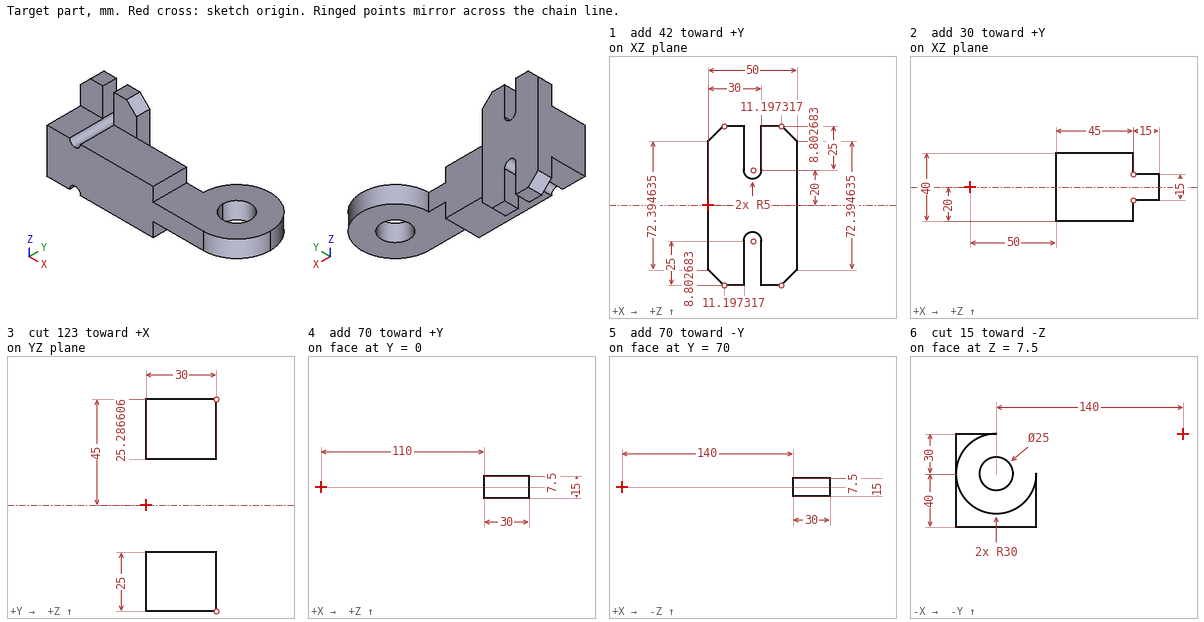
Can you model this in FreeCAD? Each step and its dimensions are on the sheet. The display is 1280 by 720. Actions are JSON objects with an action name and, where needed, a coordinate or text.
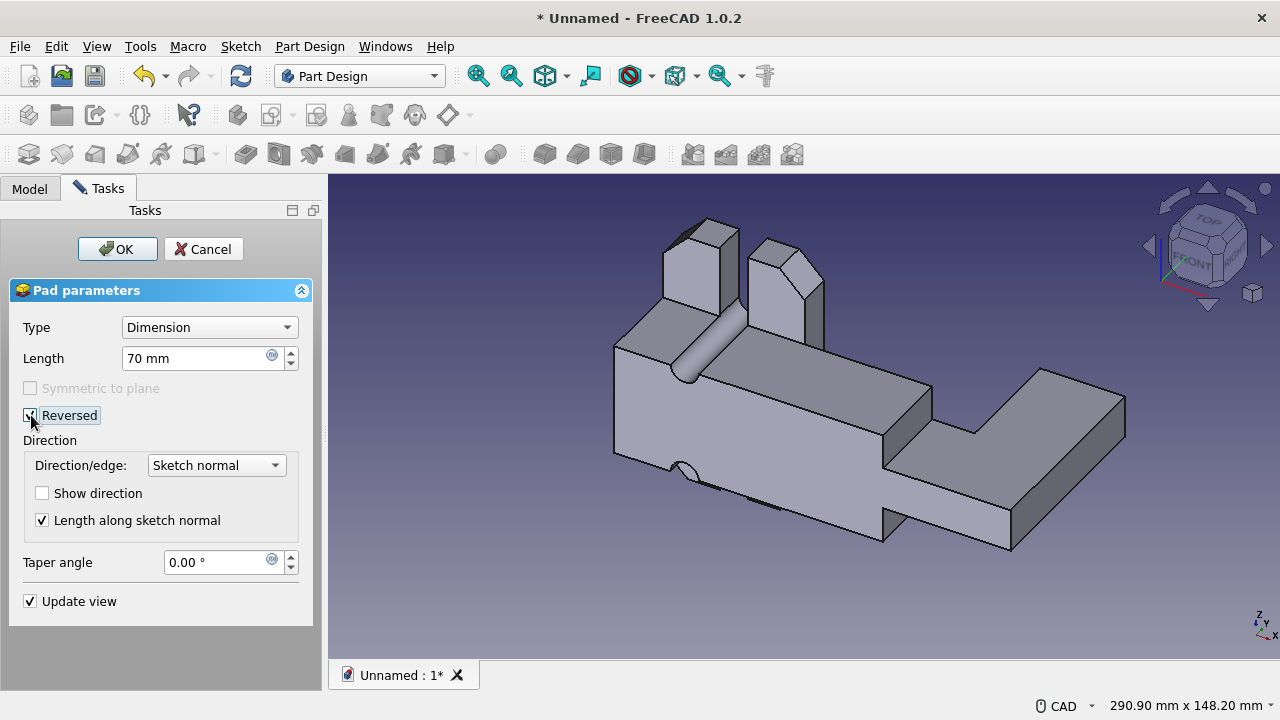
{"action": "left_click", "coordinate": [118, 249]}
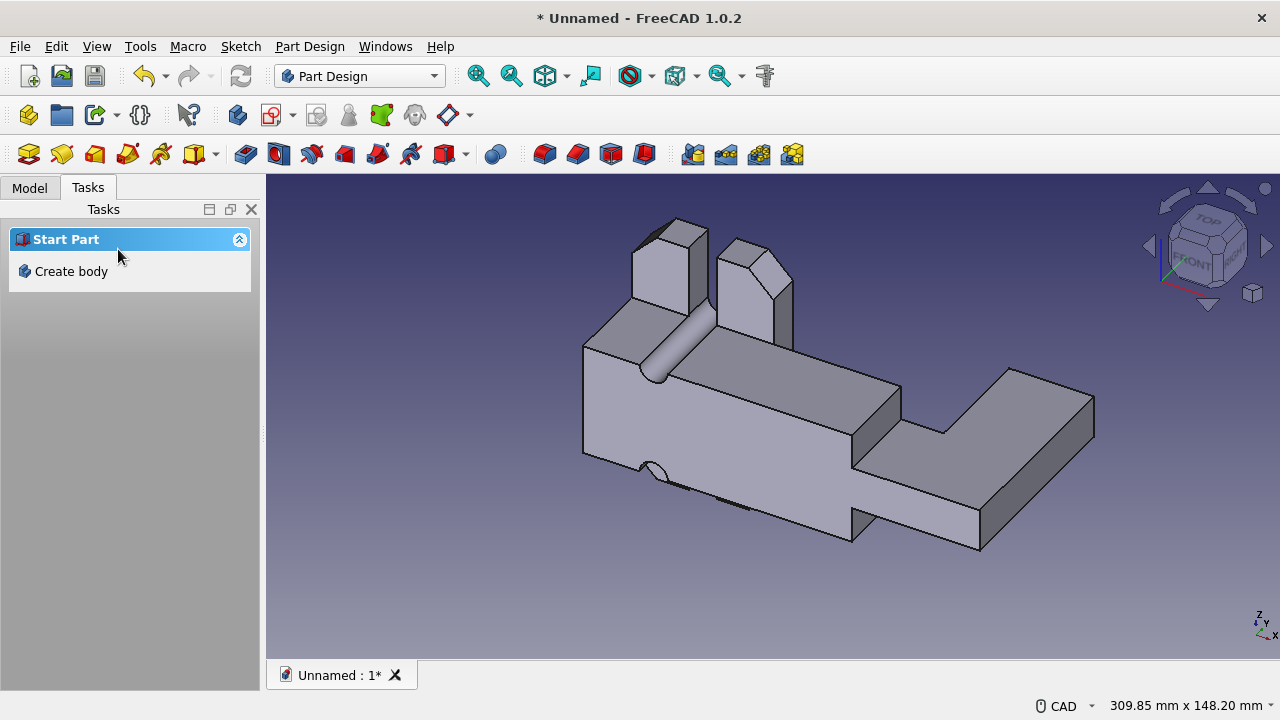
{"action": "left_click", "coordinate": [479, 76]}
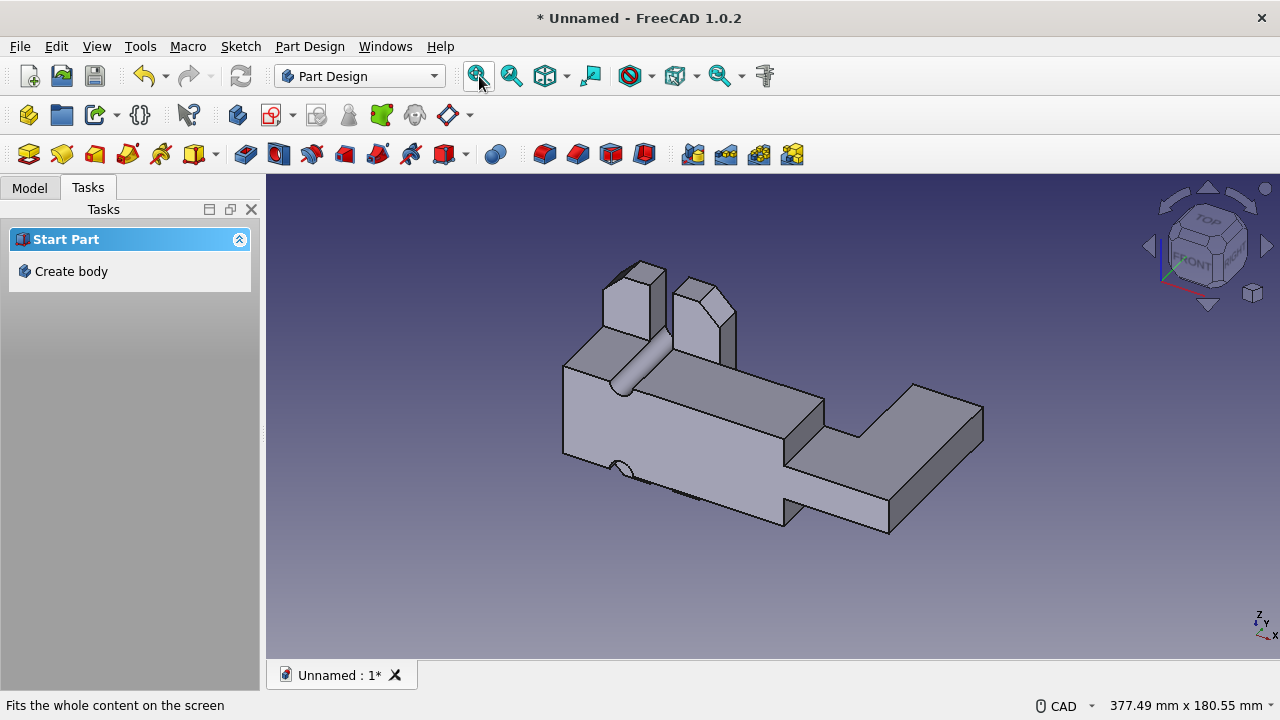
{"action": "key", "text": "4"}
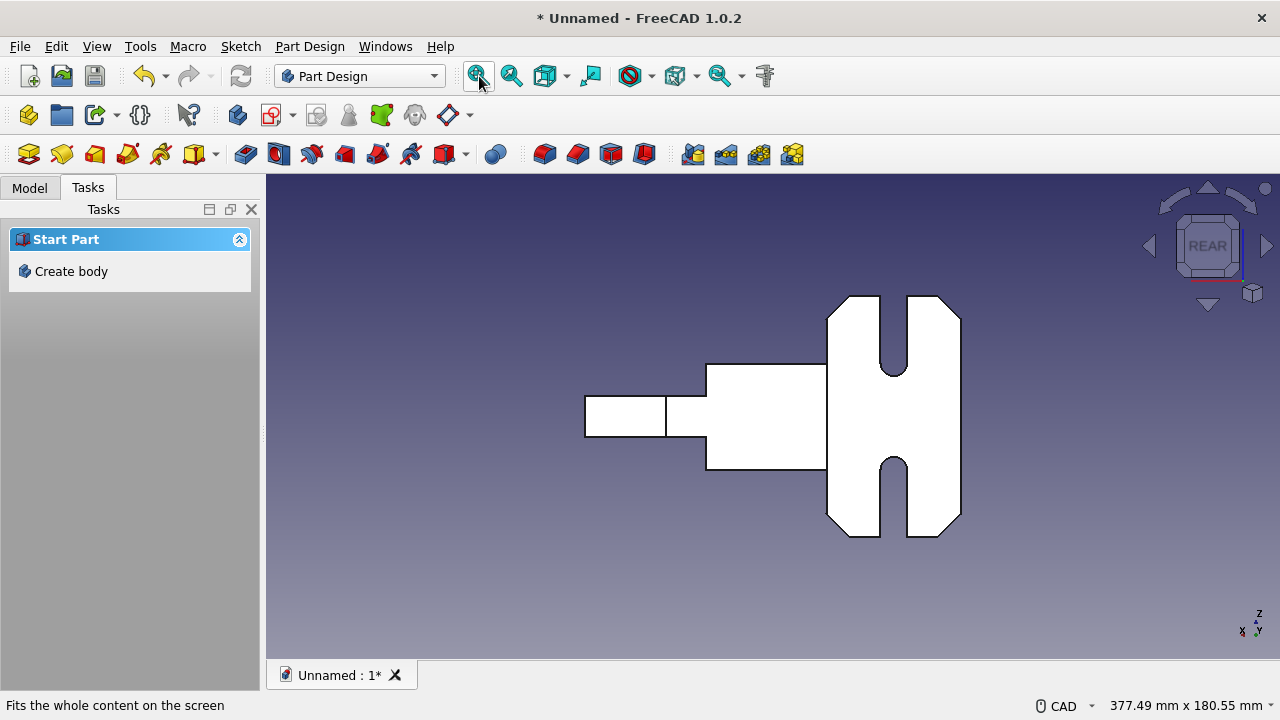
{"action": "left_click", "coordinate": [614, 416]}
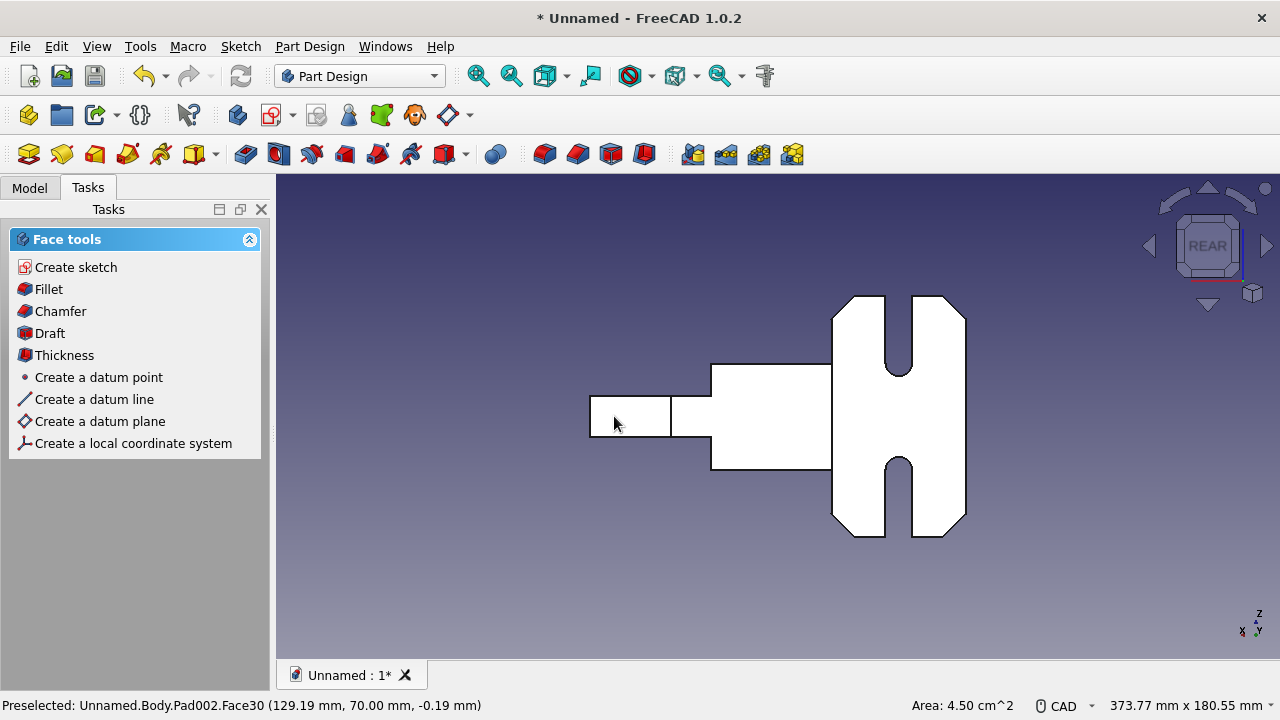
{"action": "left_click", "coordinate": [270, 116]}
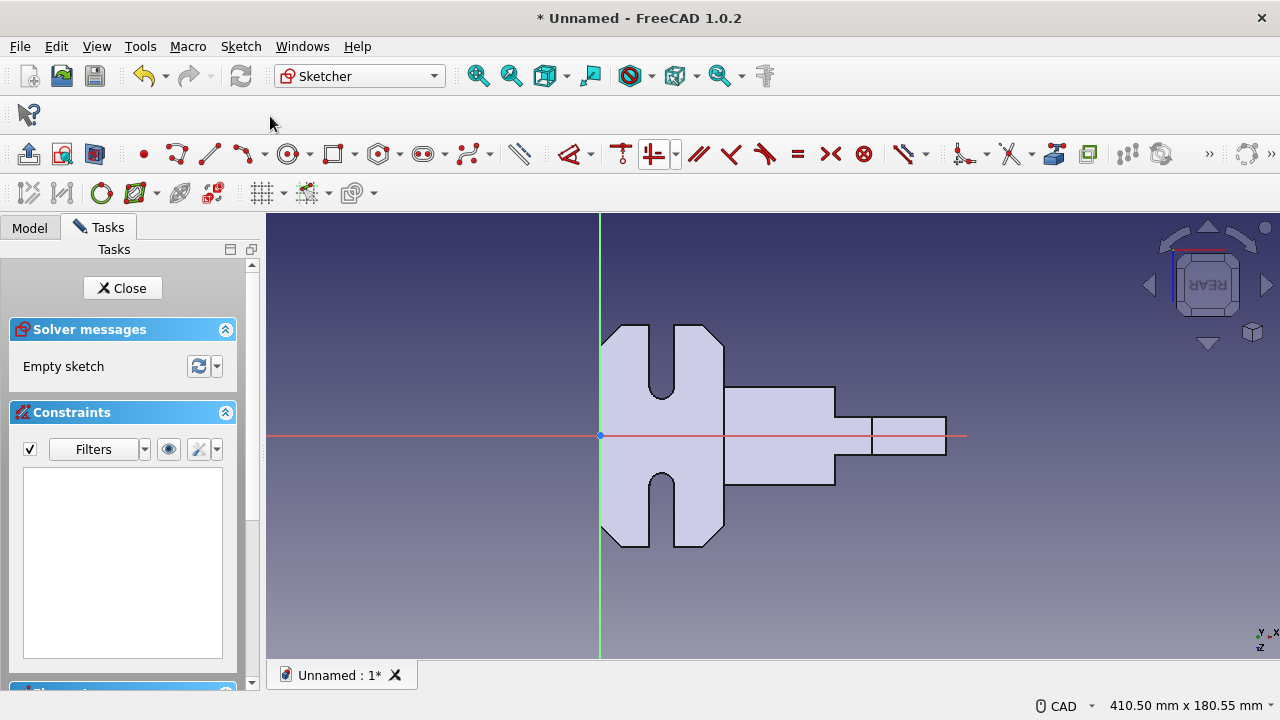
{"action": "scroll", "coordinate": [1027, 436], "scroll_direction": "up", "scroll_amount": 10}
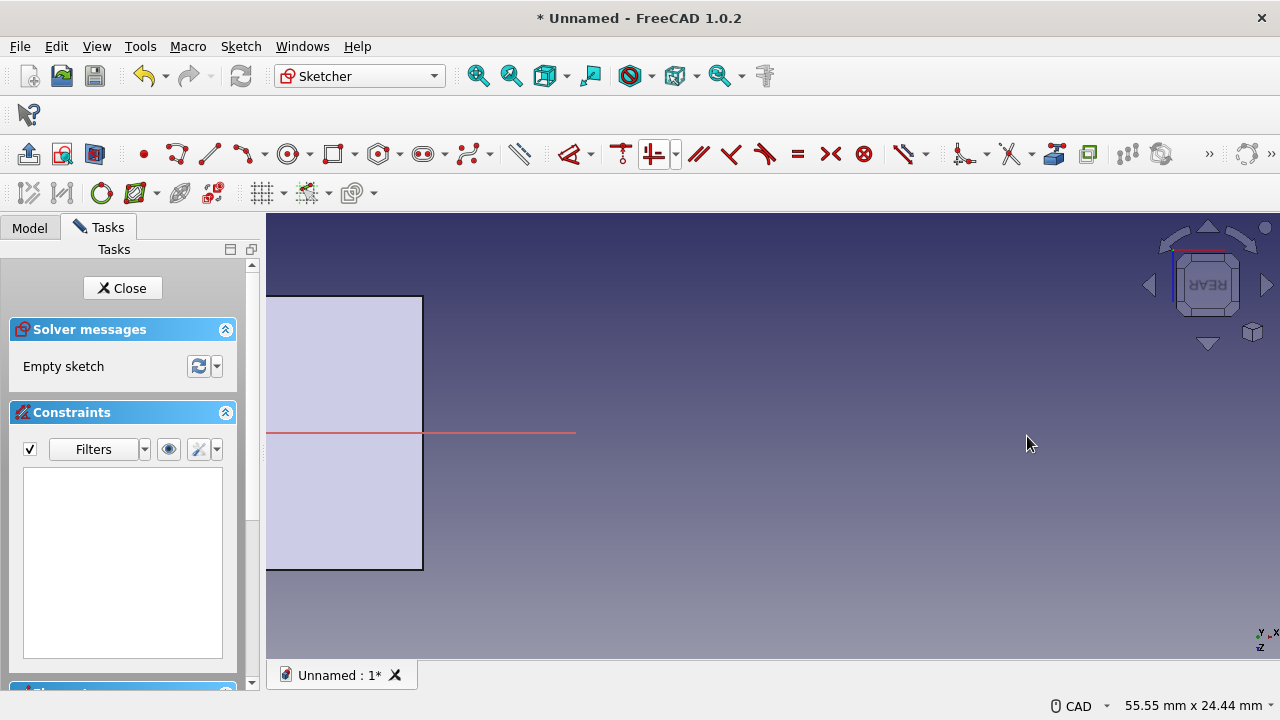
{"action": "left_click", "coordinate": [332, 154]}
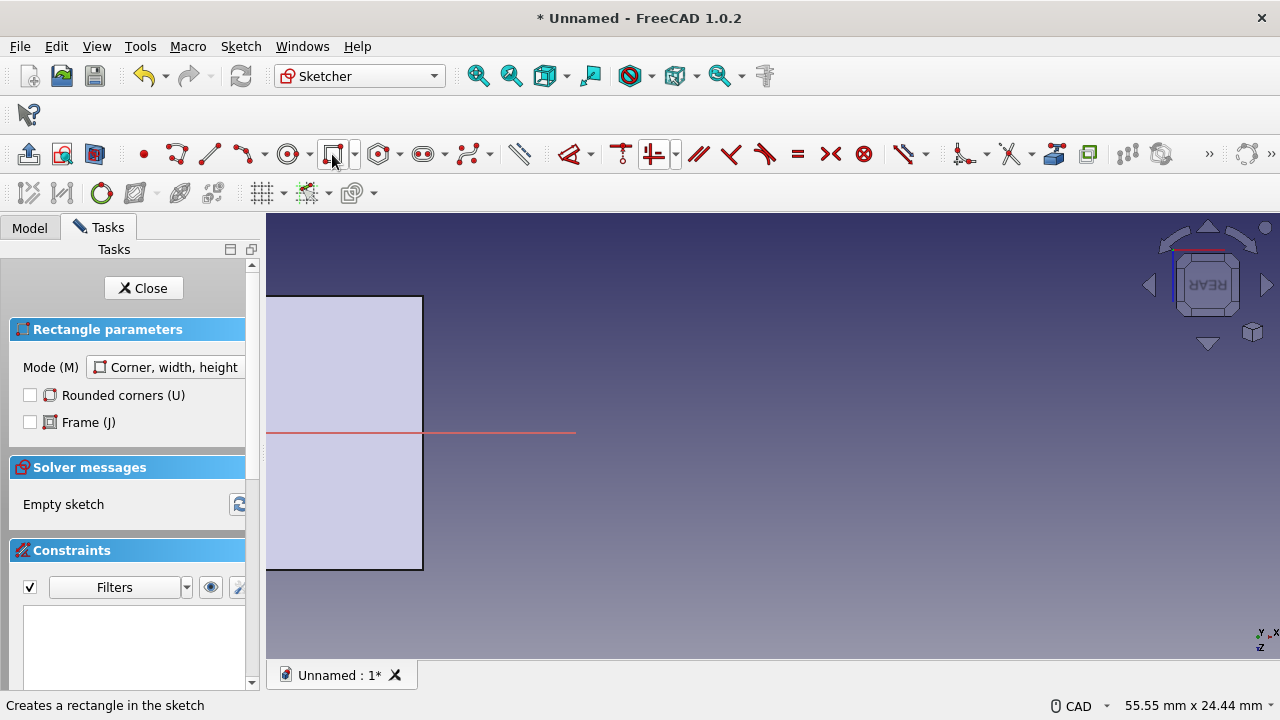
{"action": "left_click", "coordinate": [423, 296]}
{"action": "left_click", "coordinate": [971, 570]}
{"action": "key", "text": "Escape"}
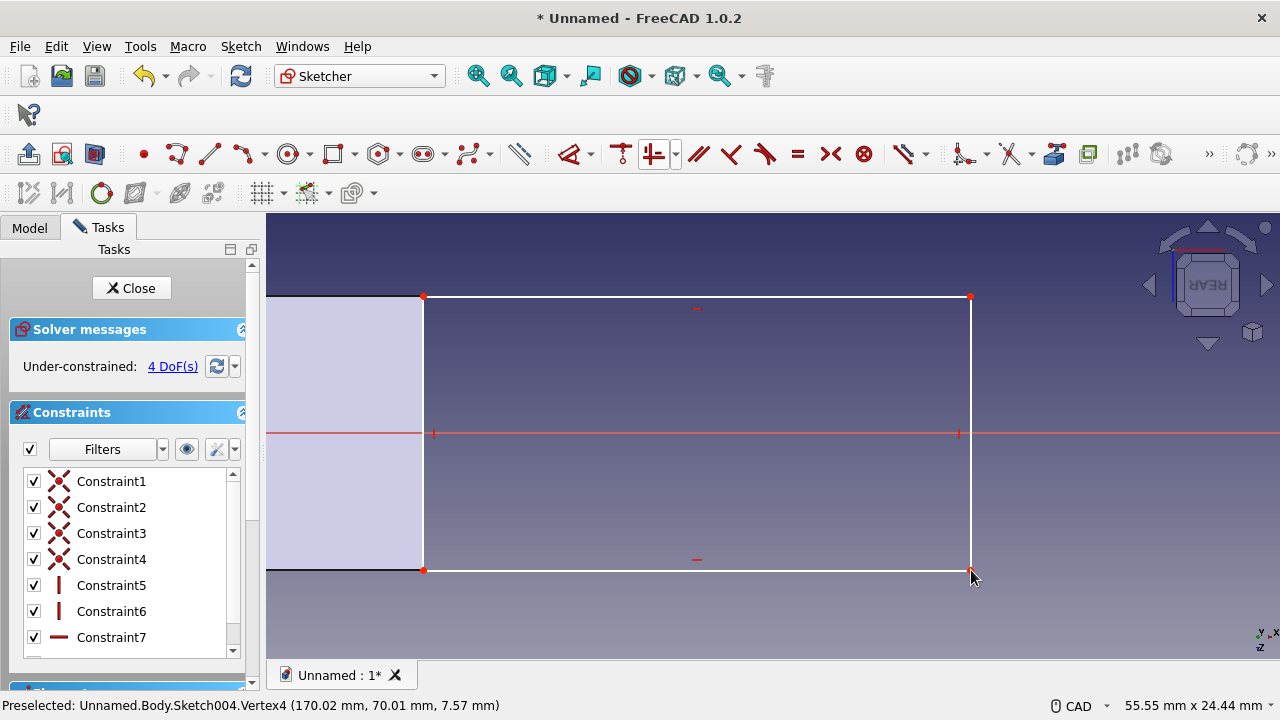
{"action": "left_click", "coordinate": [568, 154]}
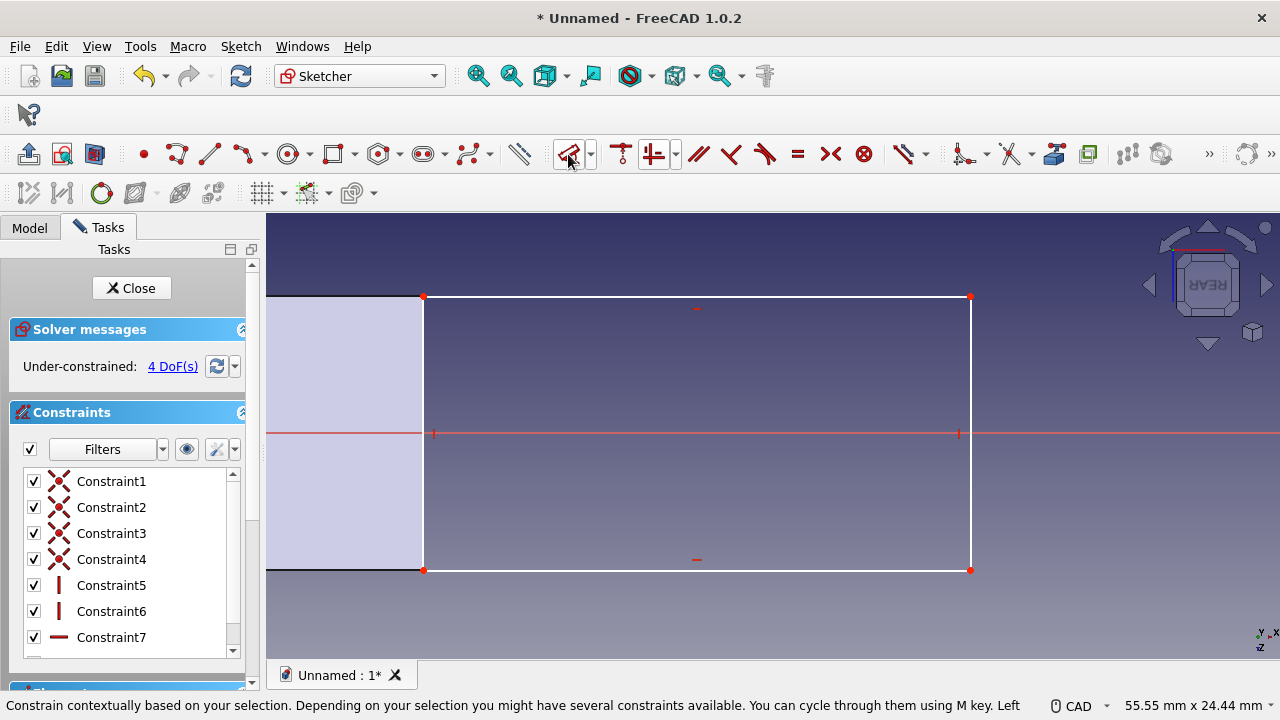
{"action": "left_click", "coordinate": [423, 379]}
{"action": "left_click", "coordinate": [389, 371]}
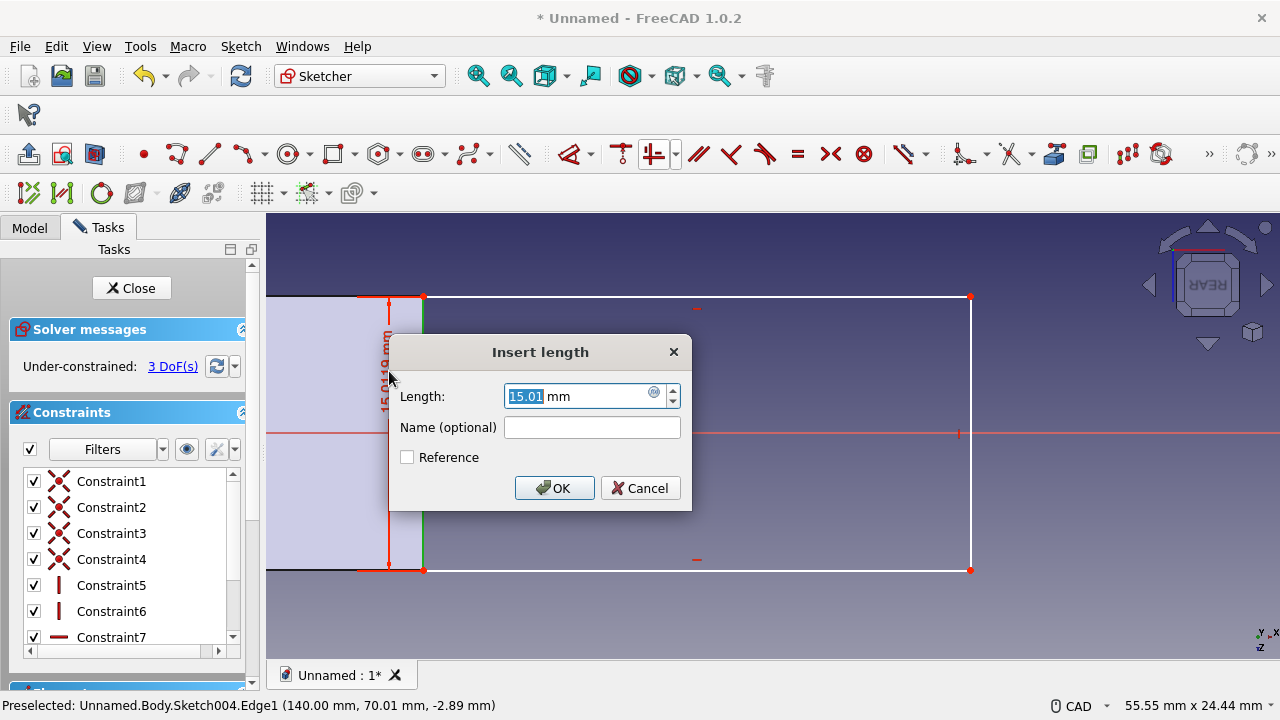
{"action": "type", "text": "15"}
{"action": "key", "text": "Return"}